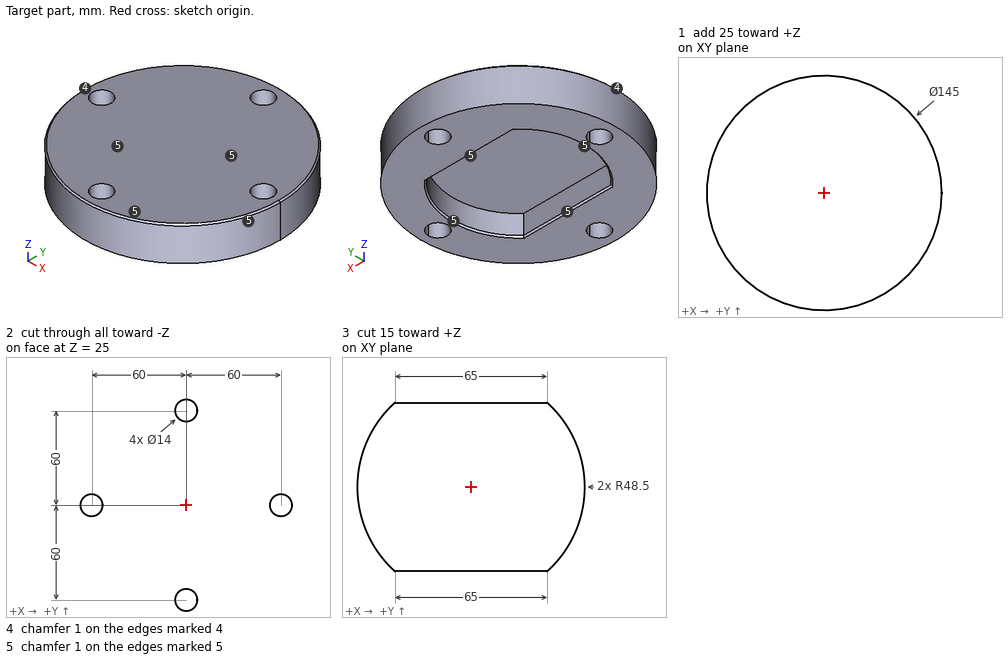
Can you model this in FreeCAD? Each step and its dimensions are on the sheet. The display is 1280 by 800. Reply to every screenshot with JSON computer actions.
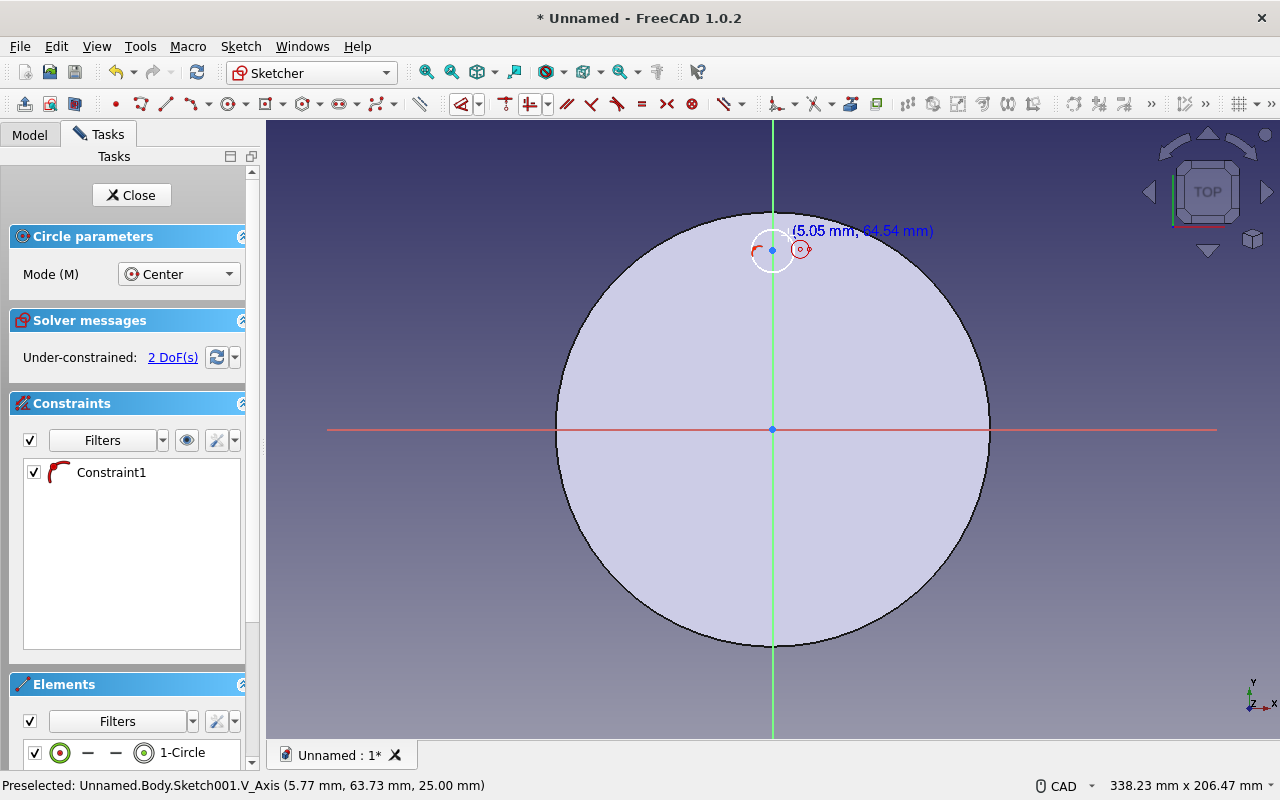
{"action": "left_click", "coordinate": [953, 430]}
{"action": "left_click", "coordinate": [968, 415]}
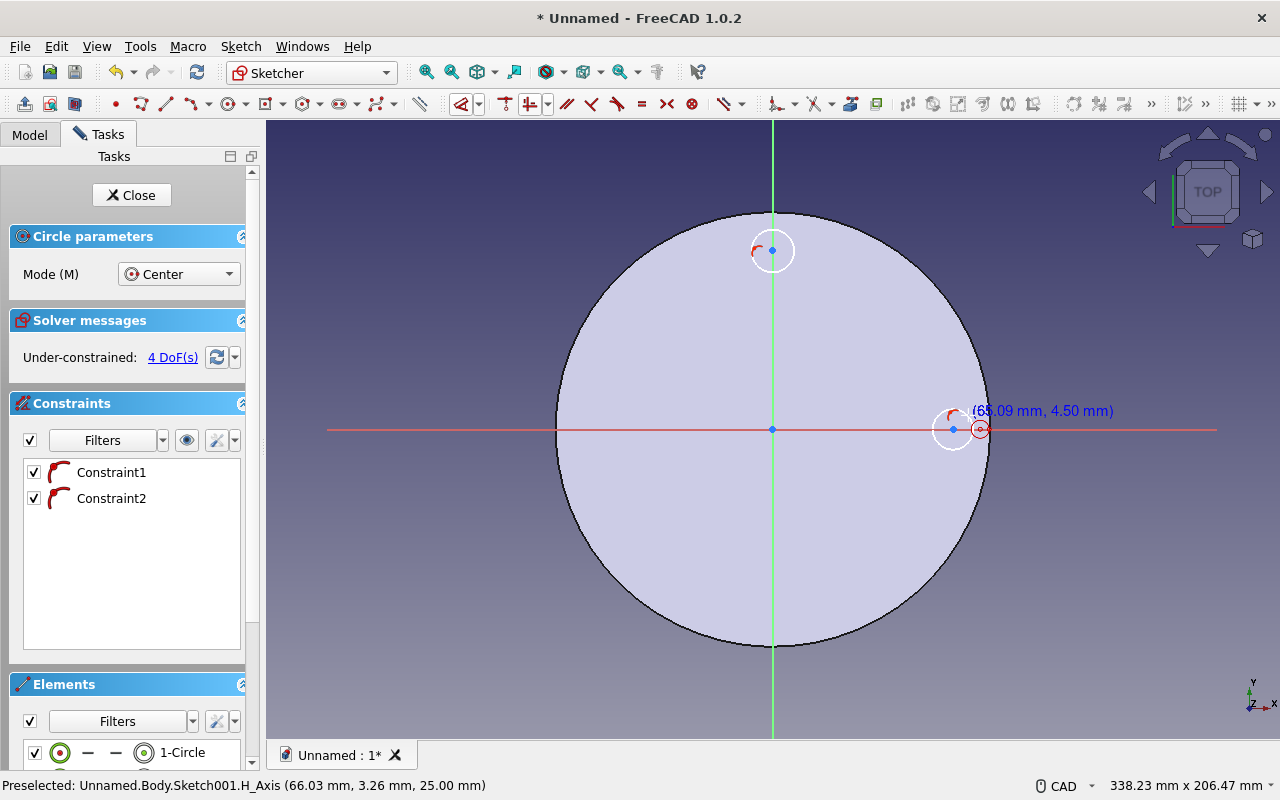
{"action": "left_click", "coordinate": [773, 609]}
{"action": "left_click", "coordinate": [788, 595]}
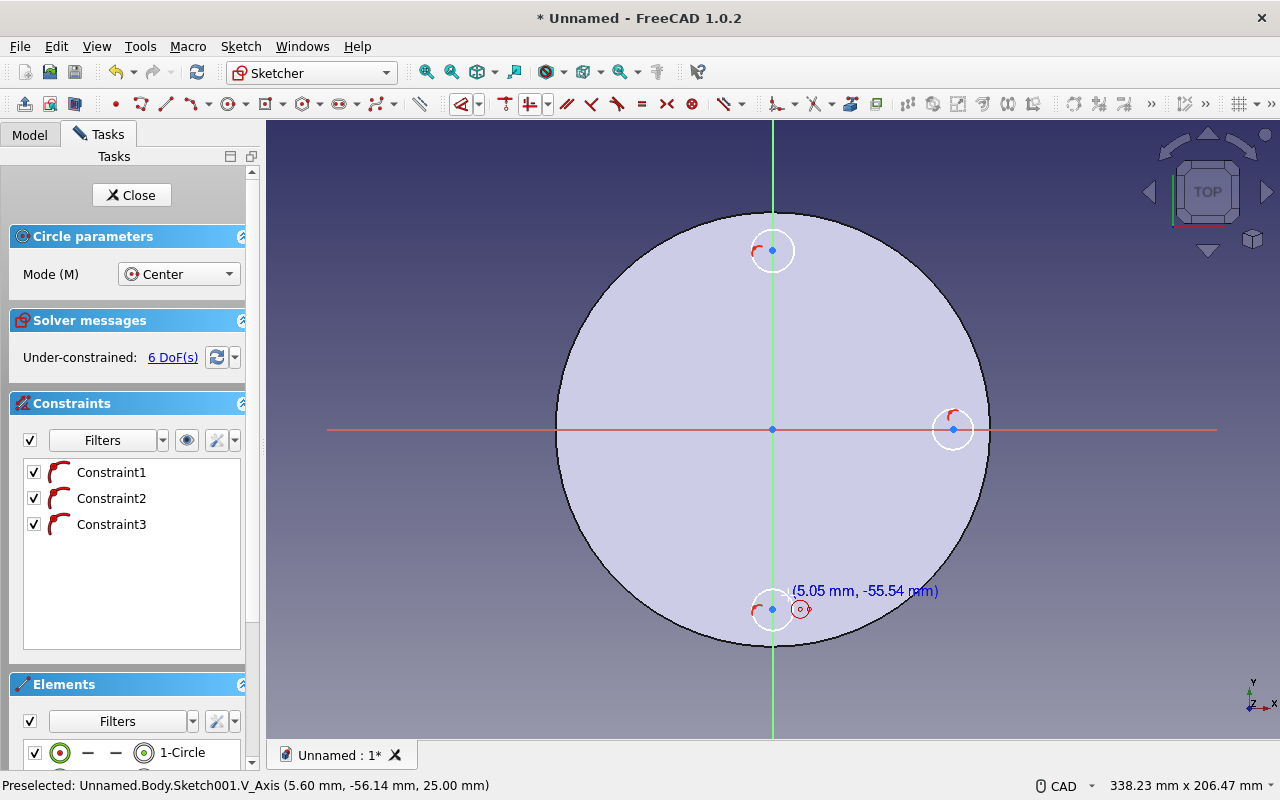
{"action": "left_click", "coordinate": [593, 430]}
{"action": "left_click", "coordinate": [608, 415]}
{"action": "key", "text": "Escape"}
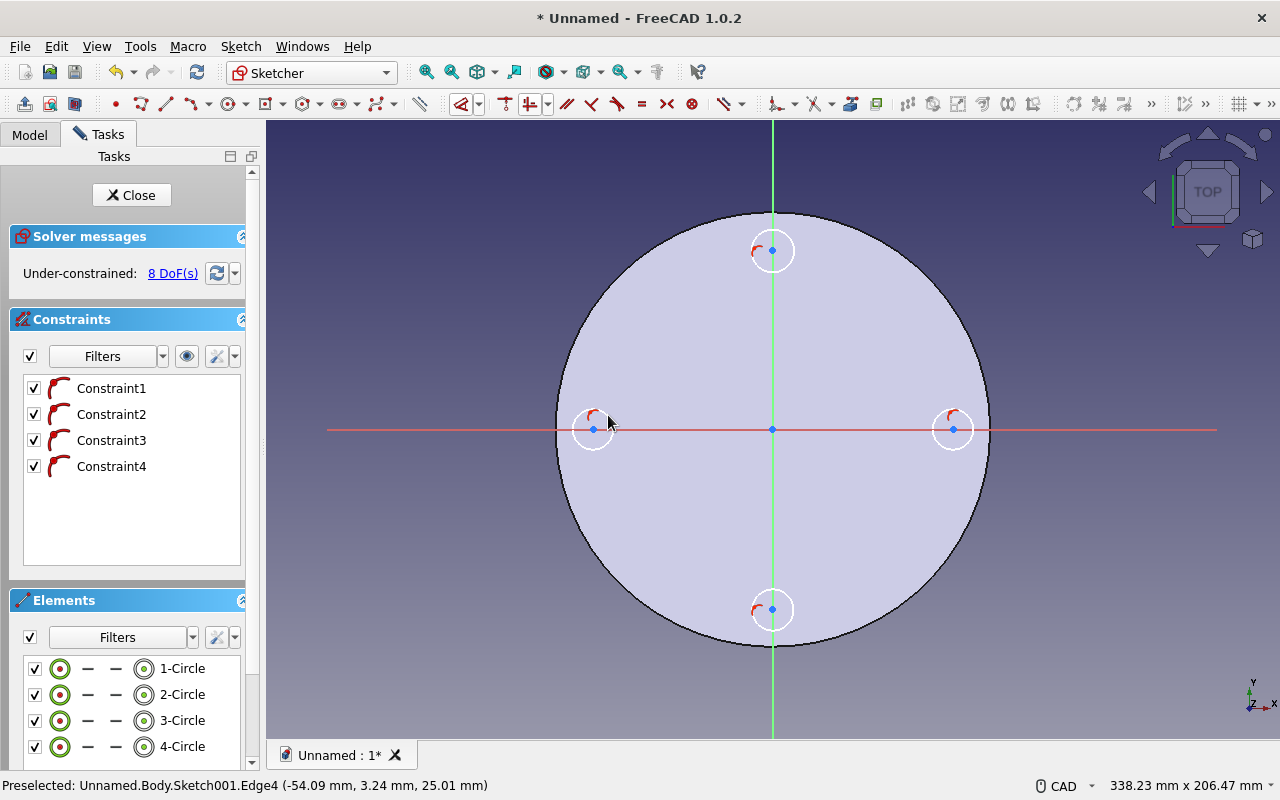
{"action": "left_click", "coordinate": [788, 236]}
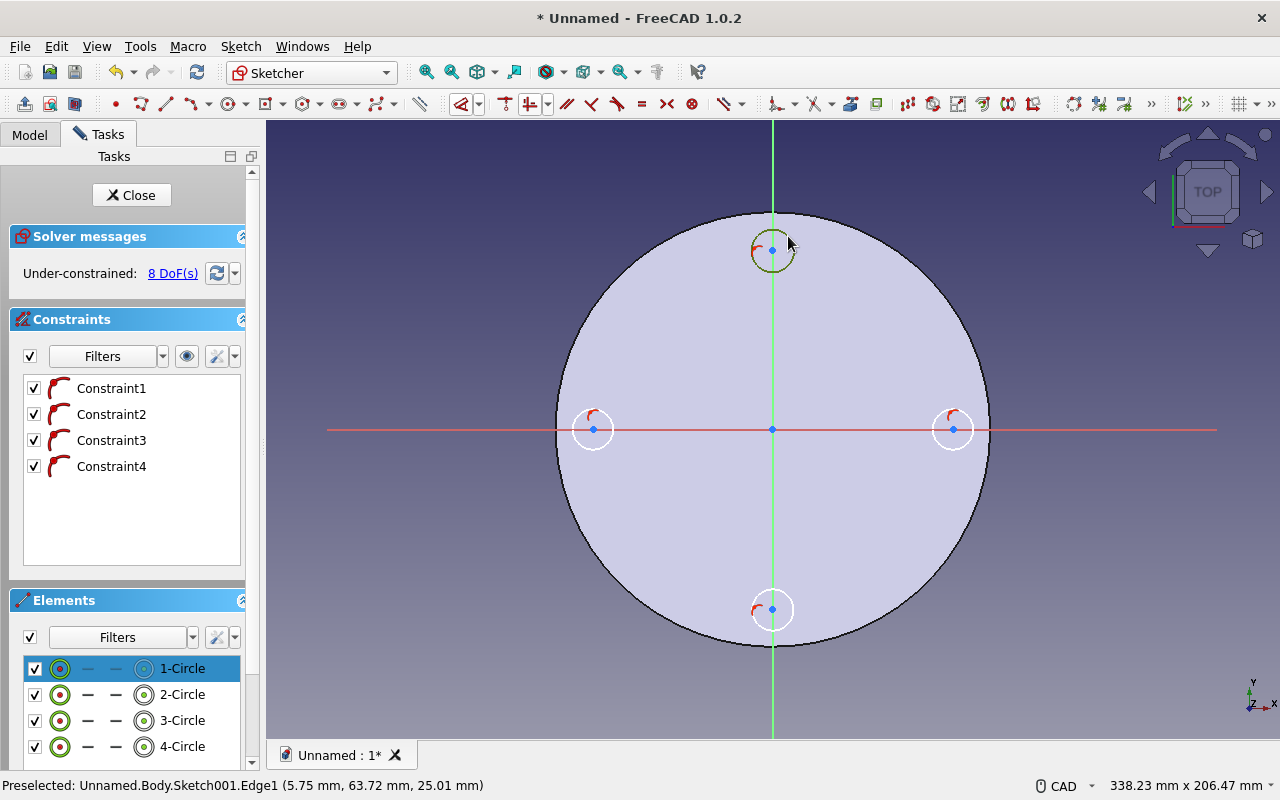
{"action": "left_click", "coordinate": [967, 415]}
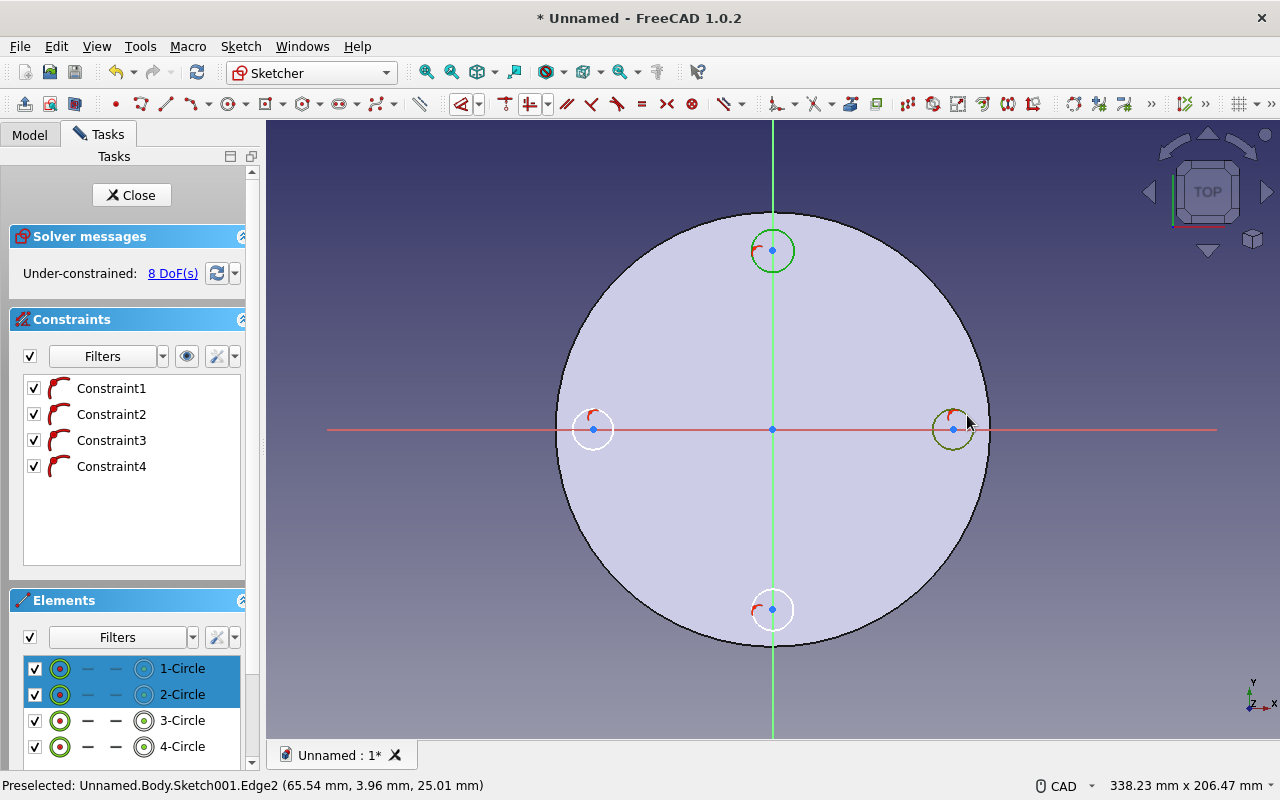
{"action": "left_click", "coordinate": [787, 595]}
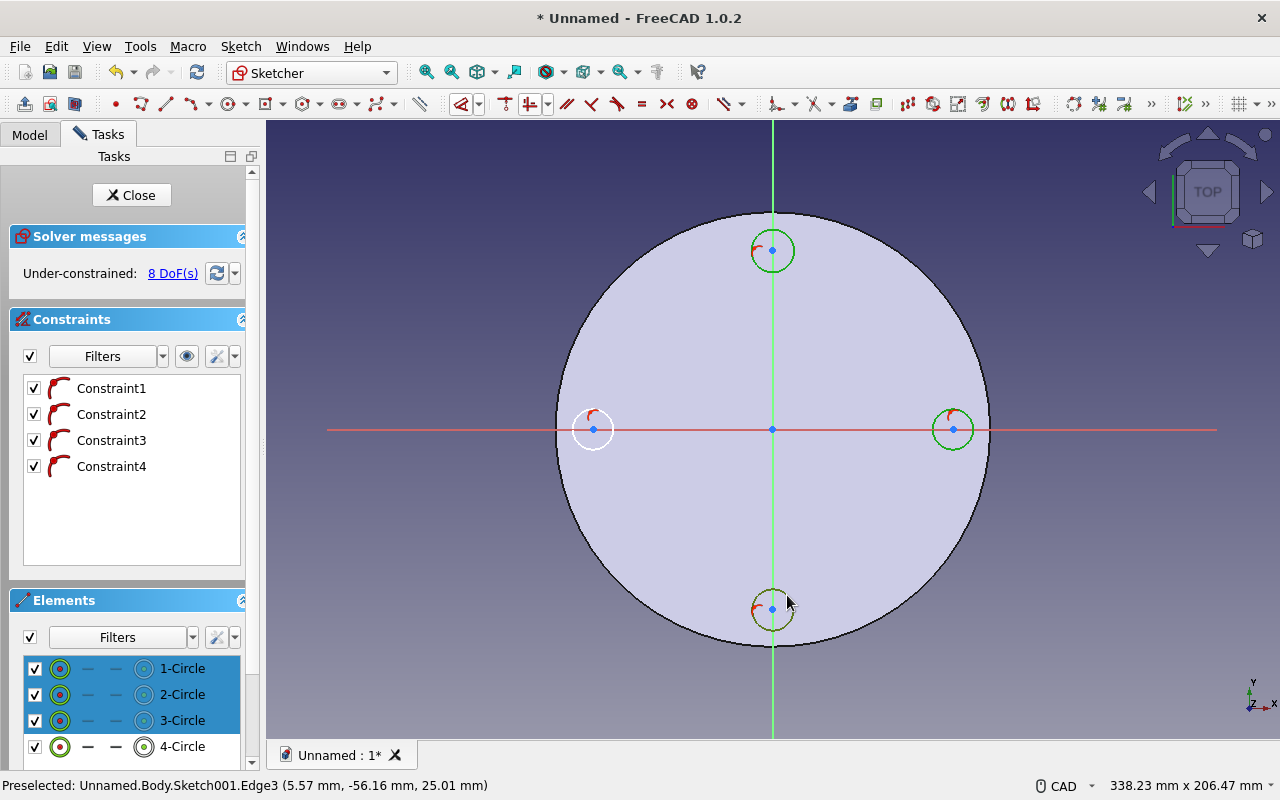
{"action": "left_click", "coordinate": [607, 415]}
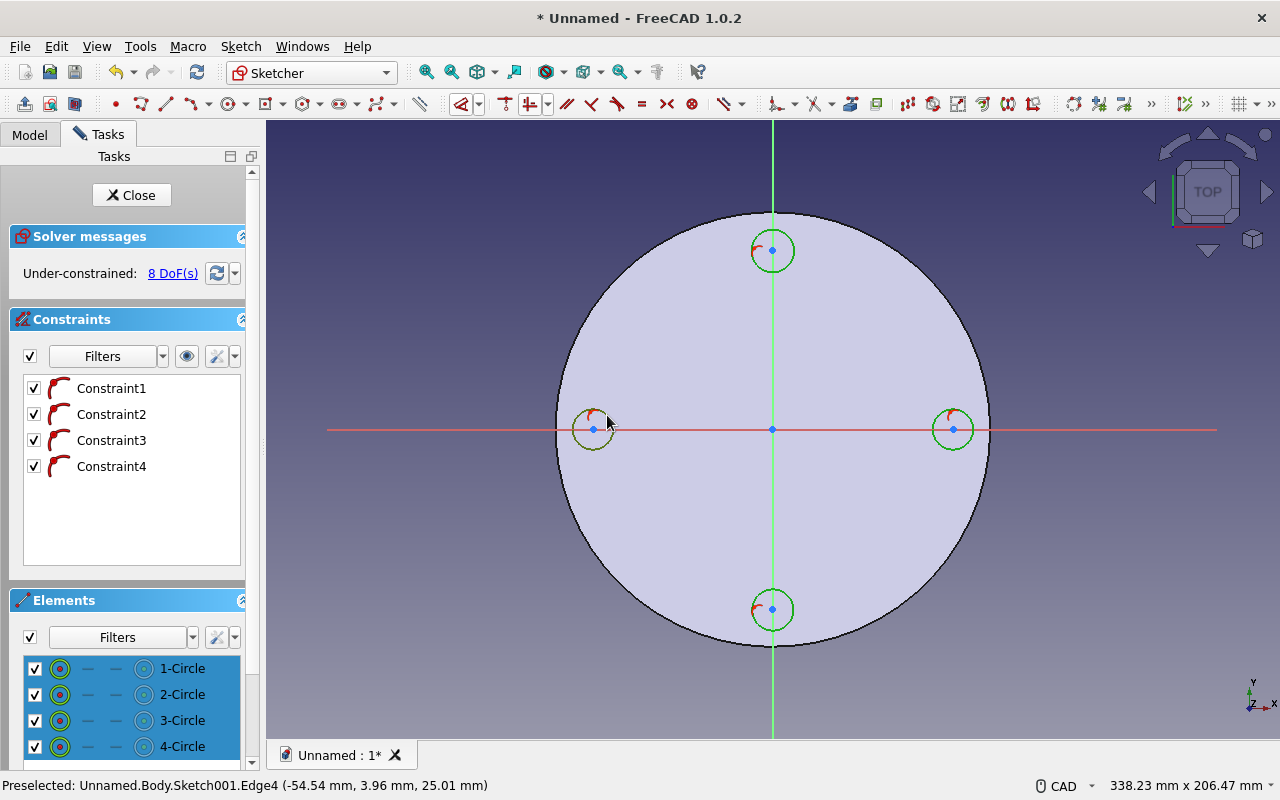
{"action": "left_click", "coordinate": [642, 104]}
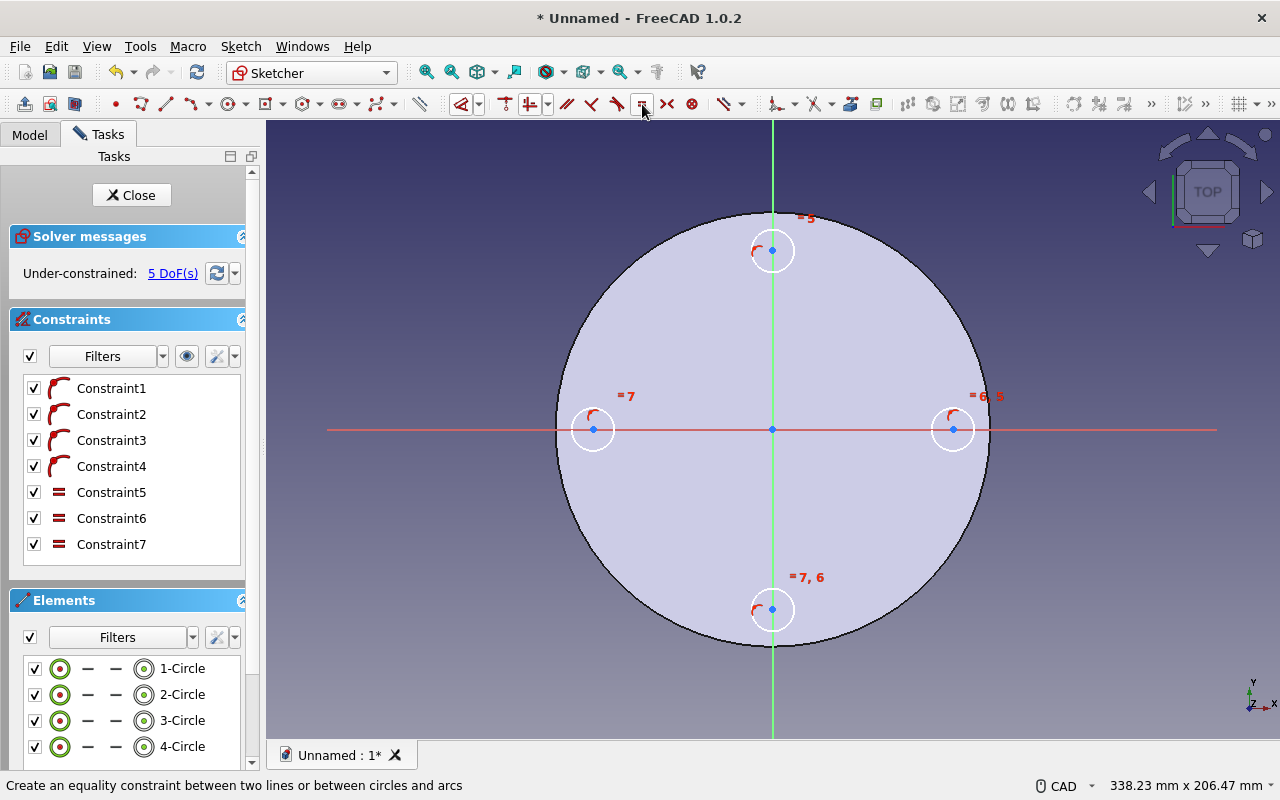
{"action": "left_click", "coordinate": [788, 236]}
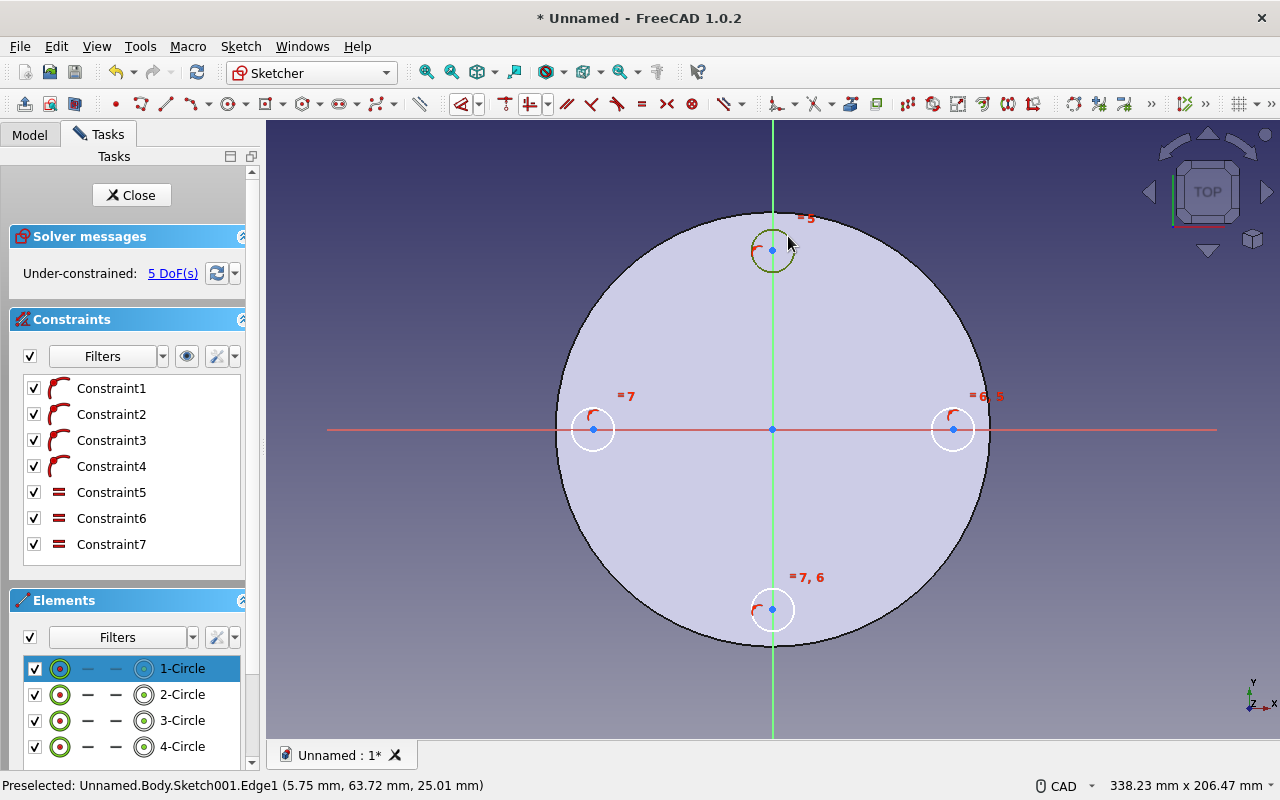
{"action": "left_click", "coordinate": [478, 104]}